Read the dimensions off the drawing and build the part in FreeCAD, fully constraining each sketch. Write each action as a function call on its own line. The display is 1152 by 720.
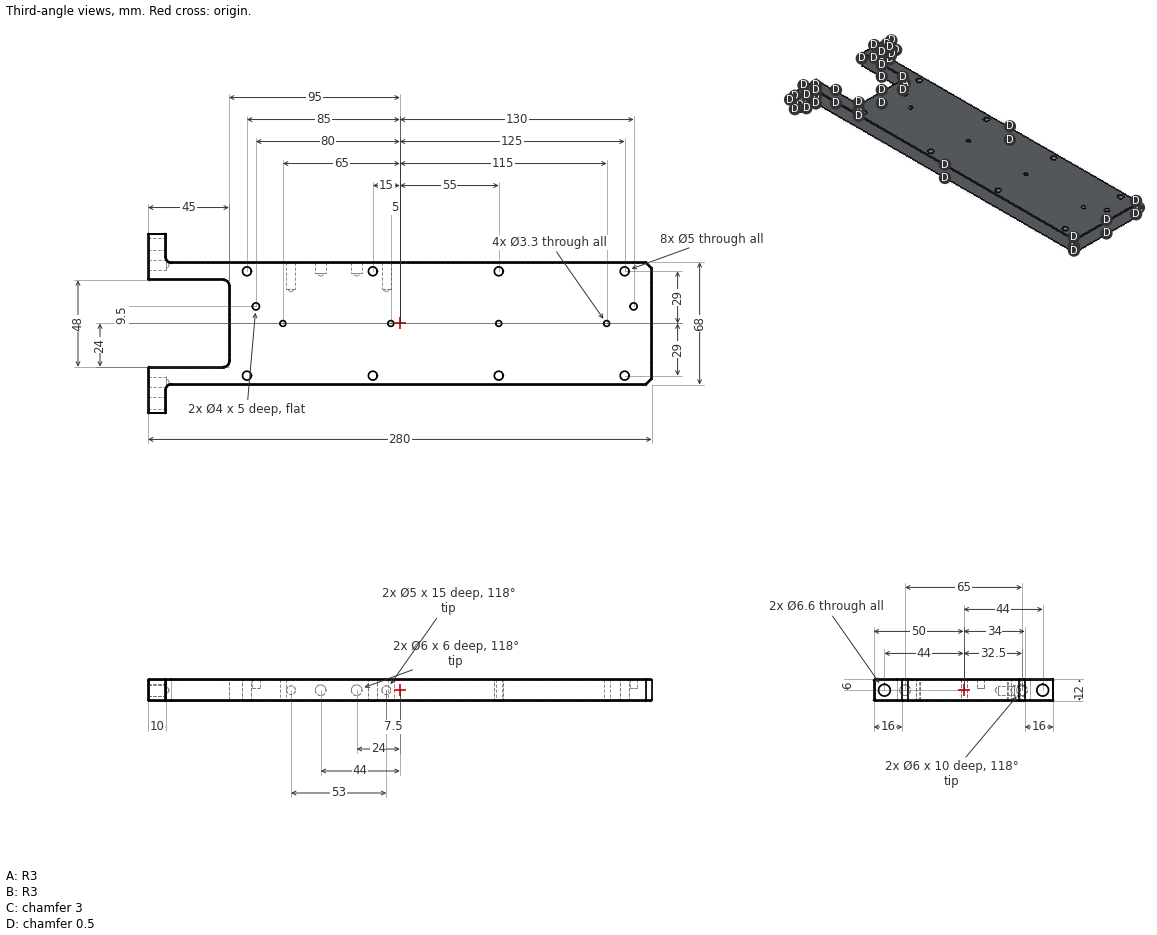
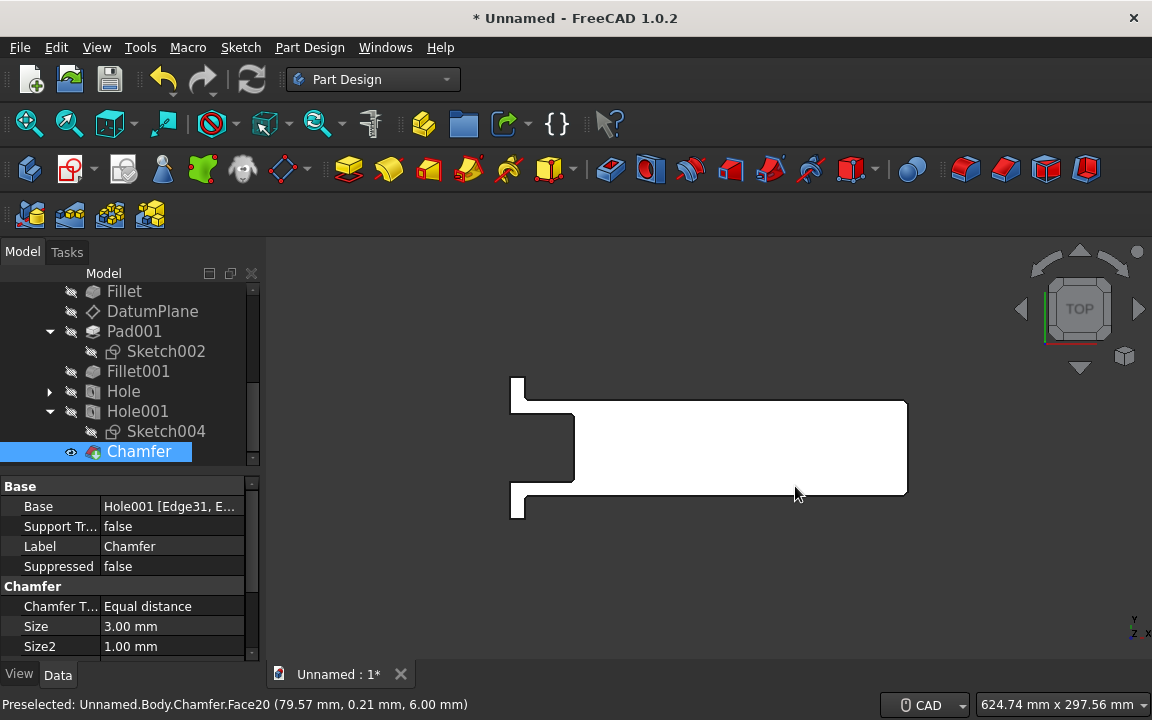
key(v)
key(f)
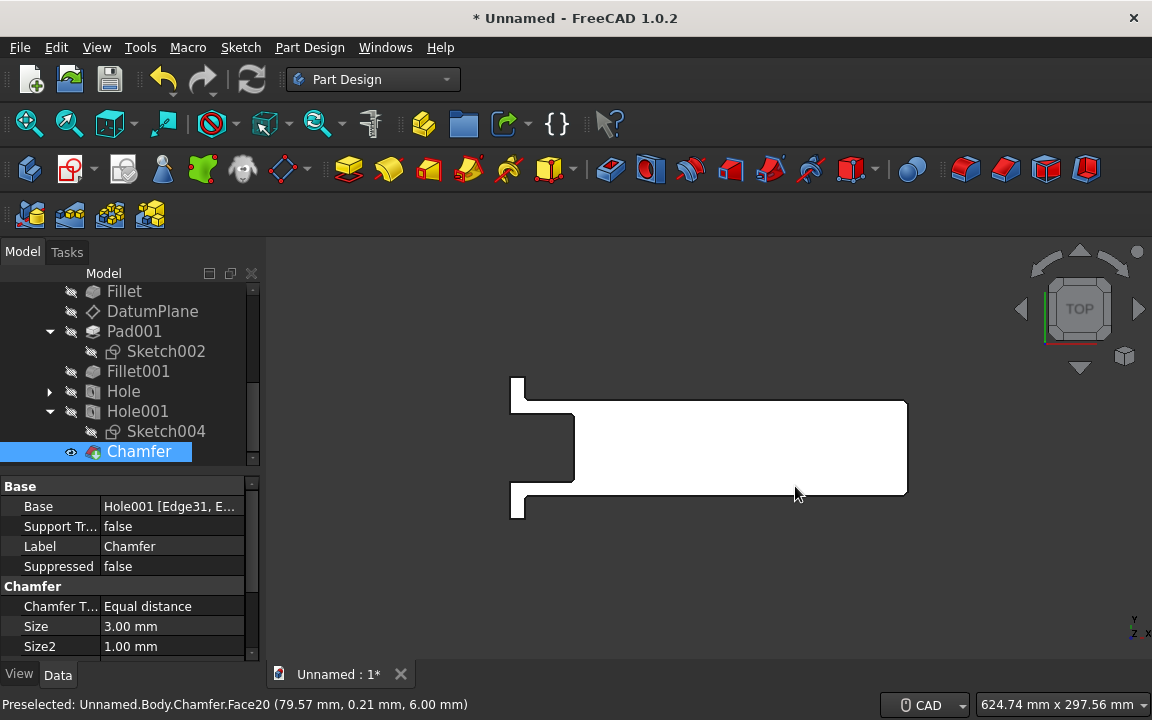
key(1)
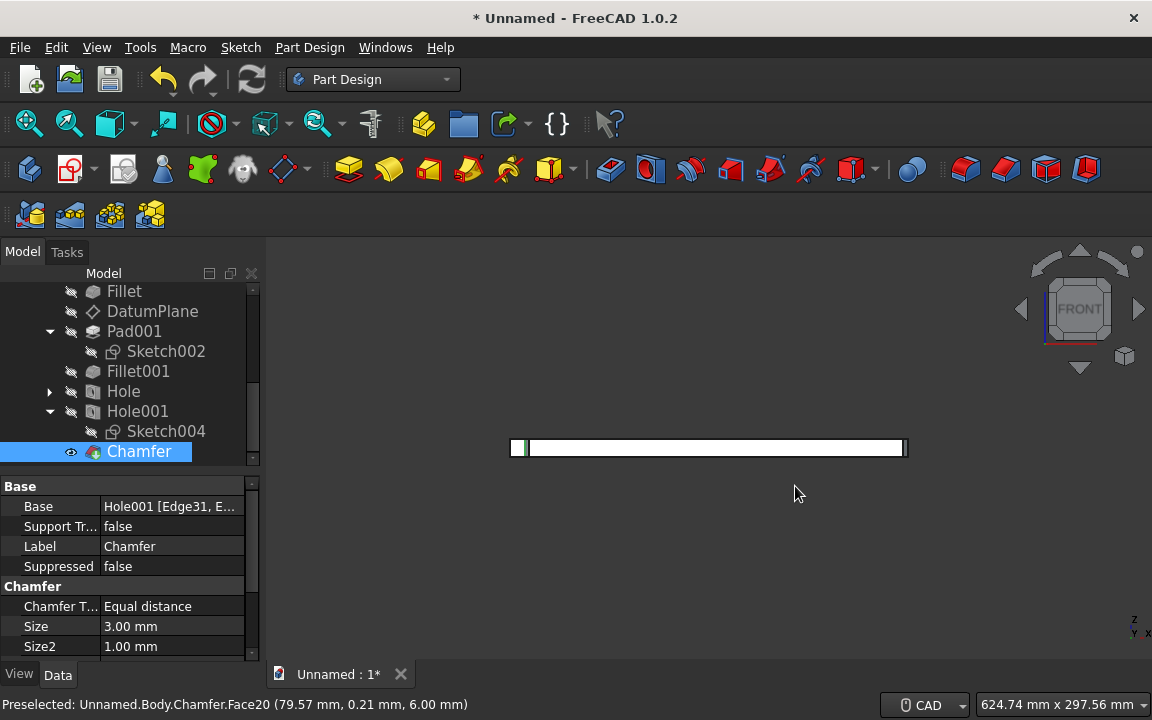
key(v)
key(f)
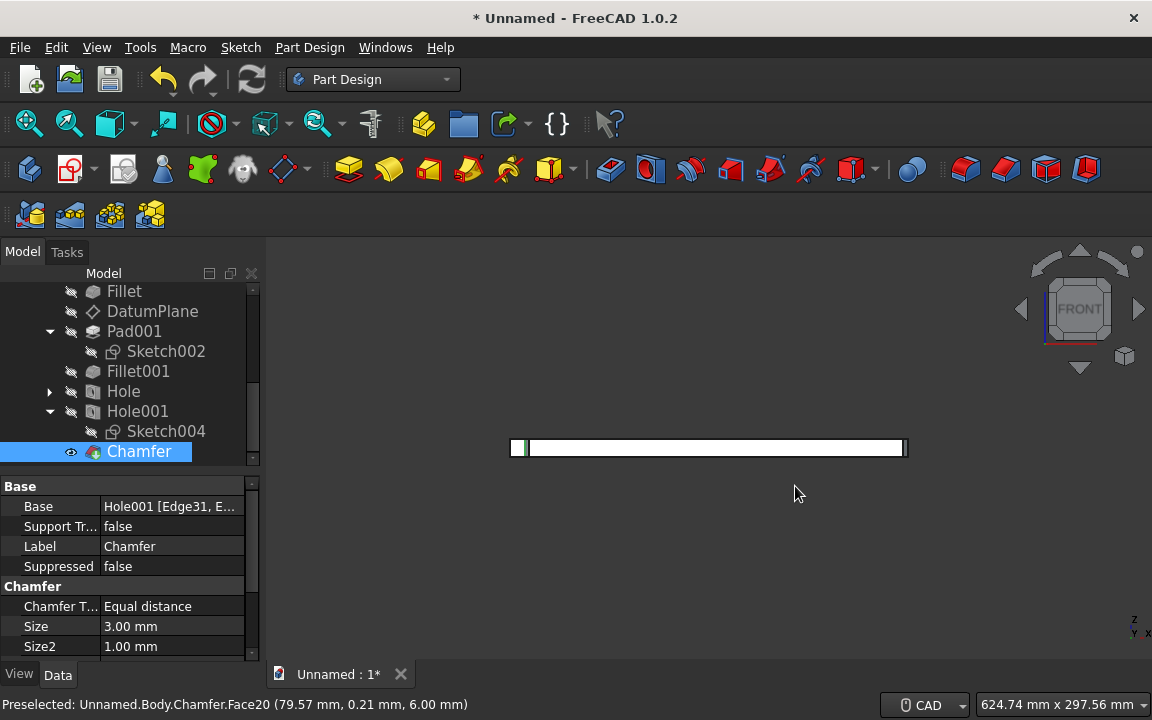
click(510, 447, ctrl)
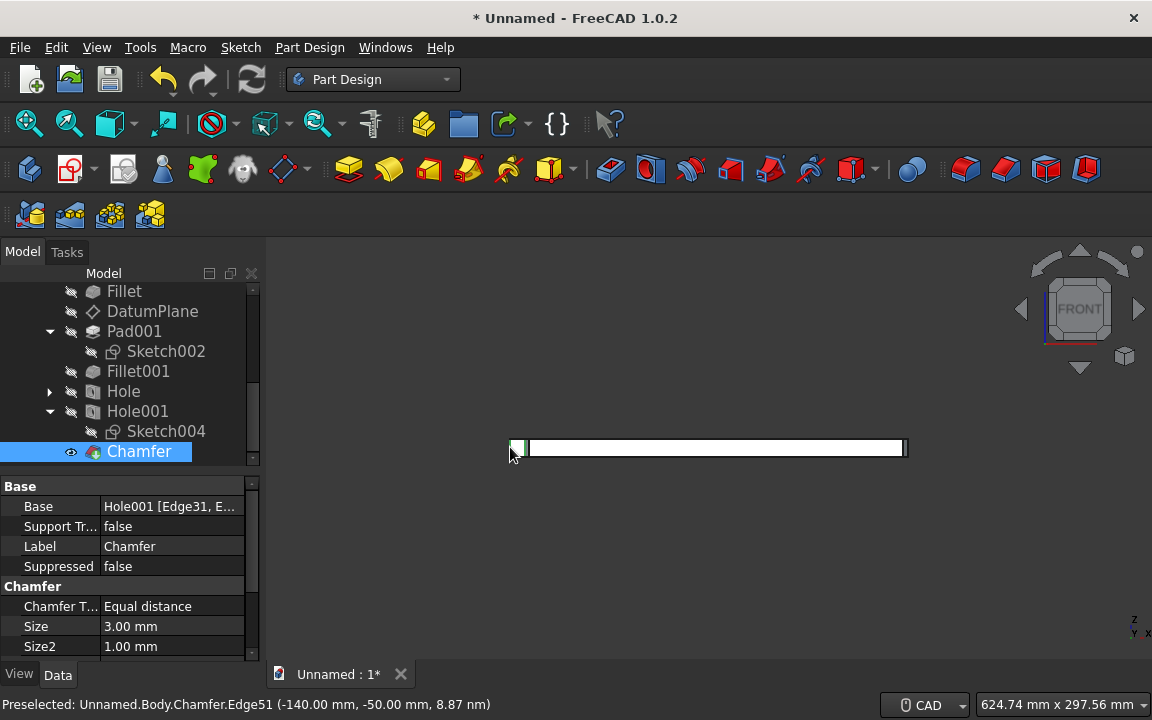
key(3)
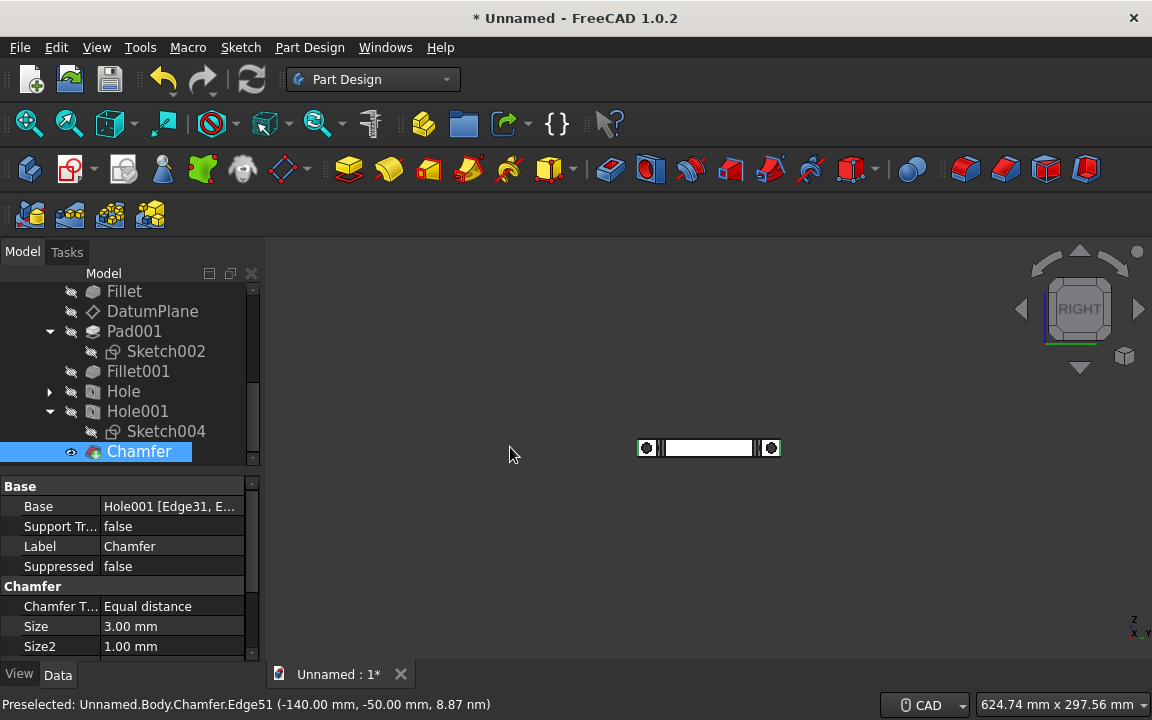
click(30, 124)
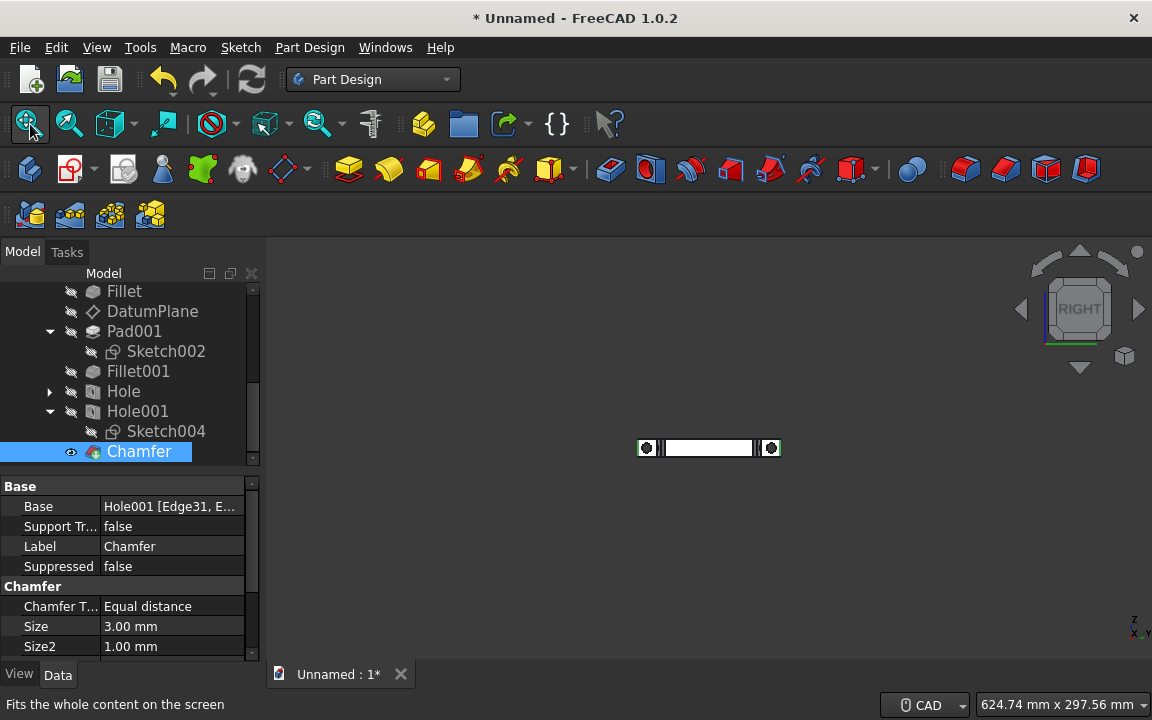
key(5)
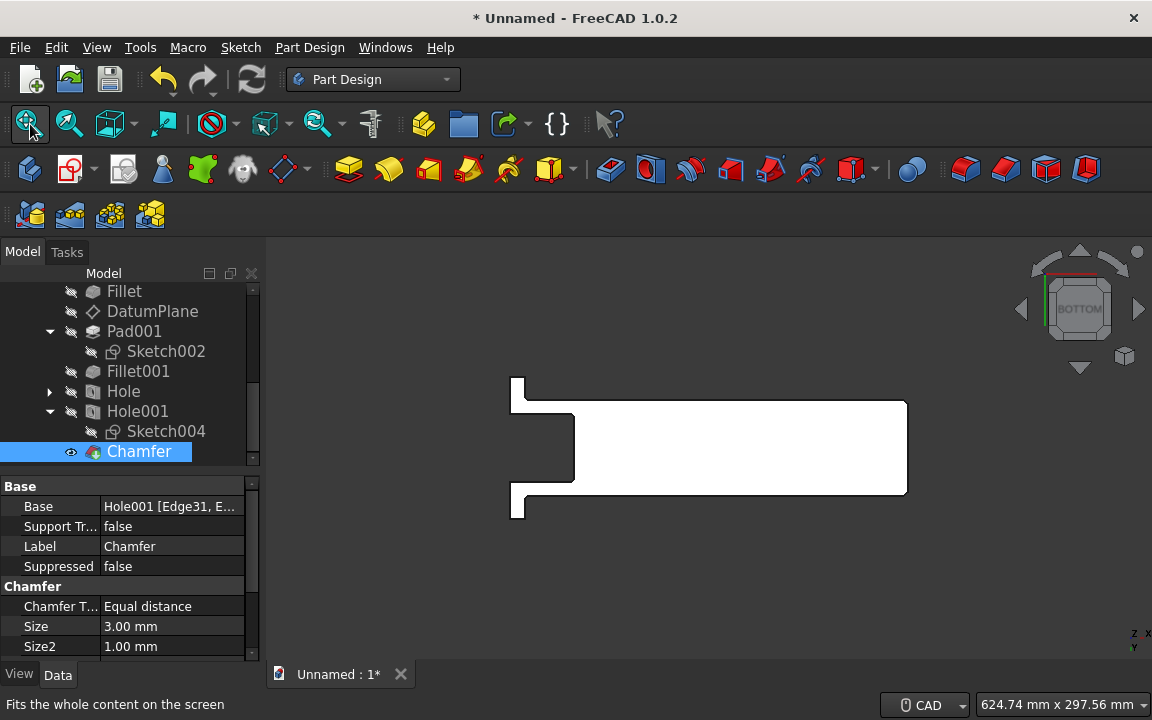
key(v)
key(f)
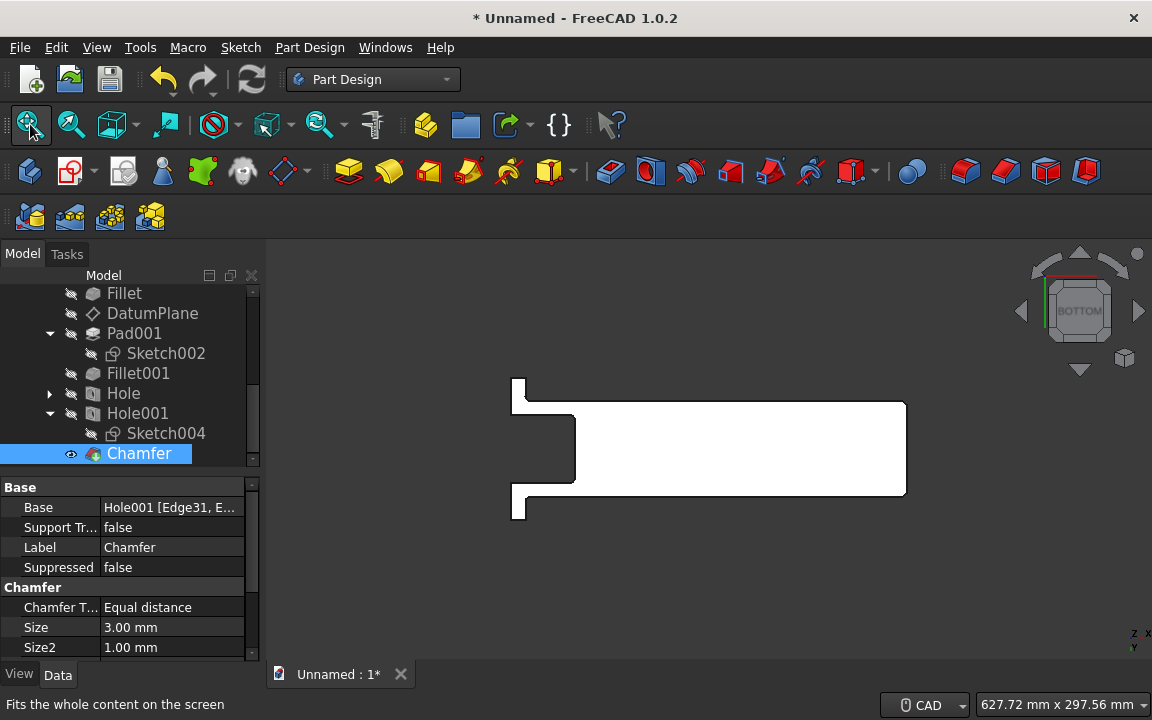
click(822, 448, ctrl)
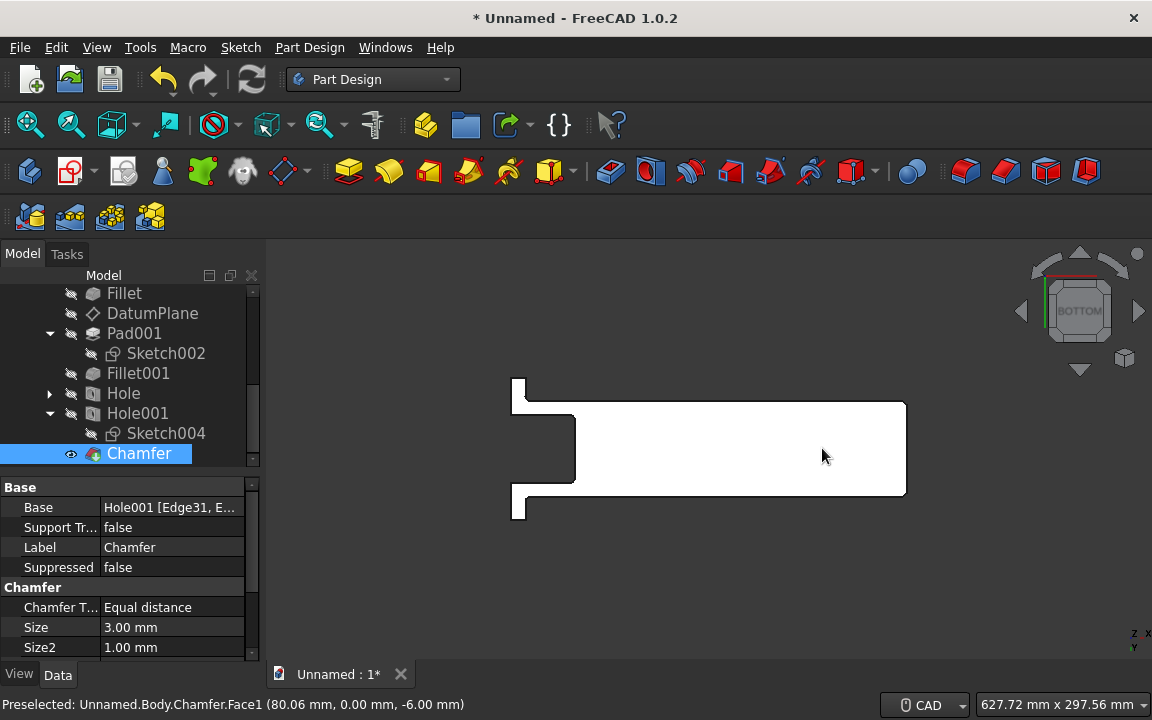
scroll(511, 482, up, 5)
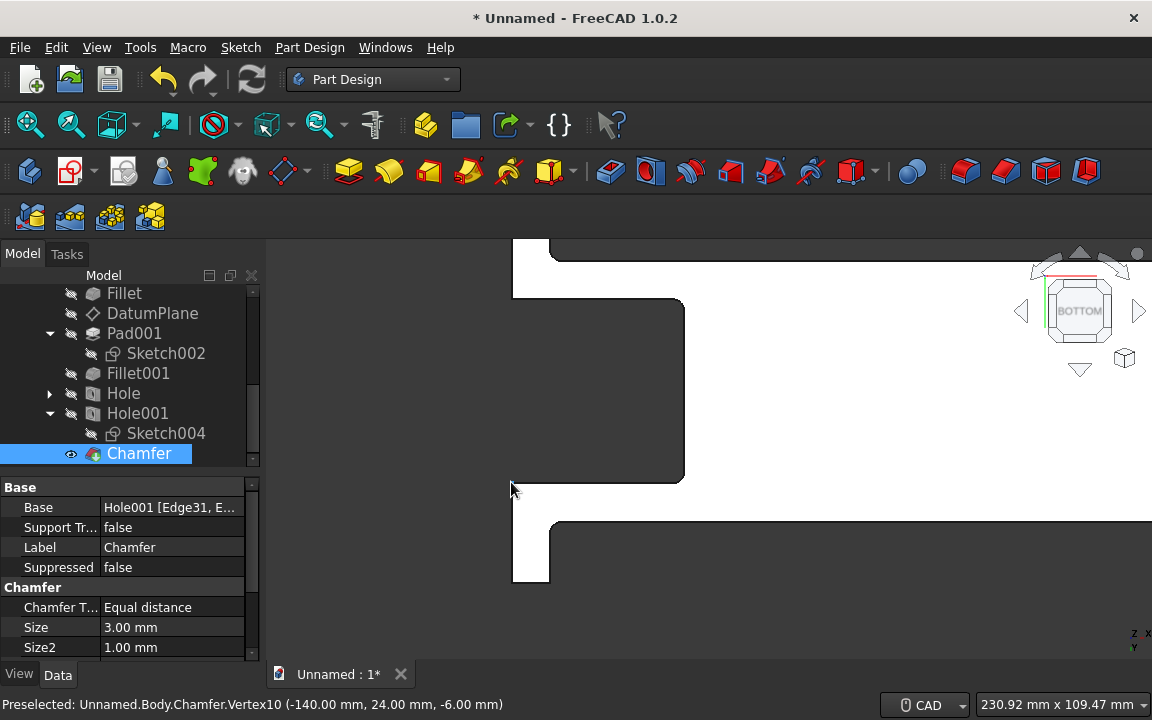
key(v)
key(f)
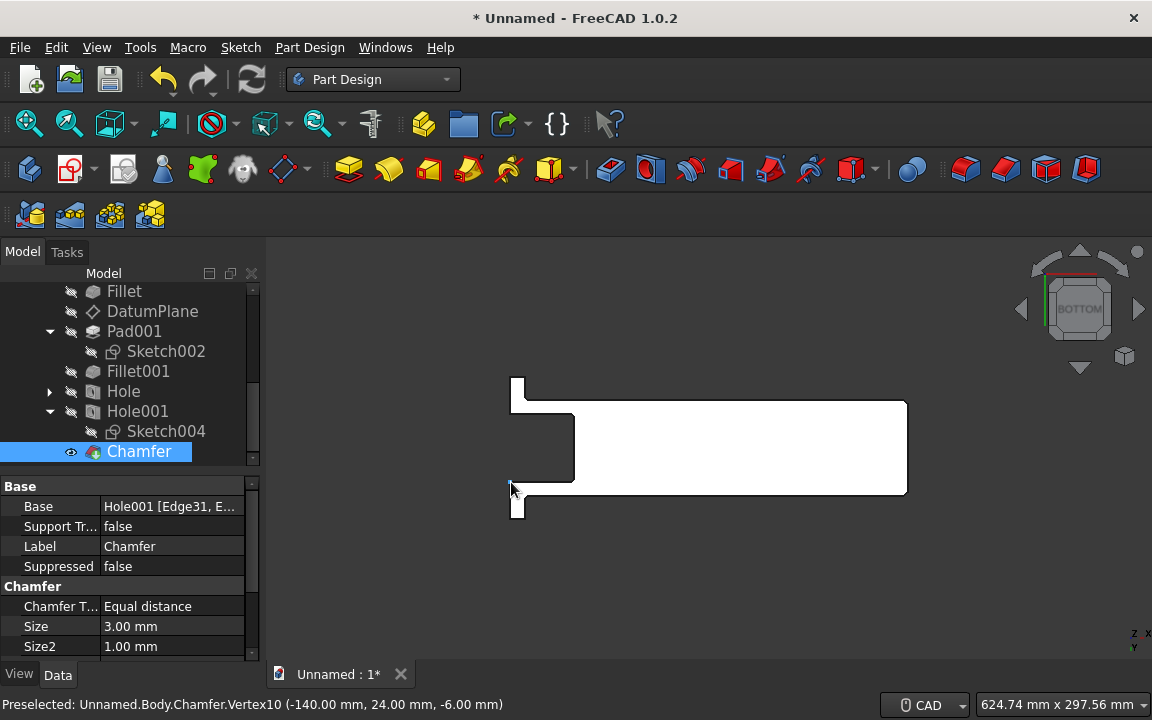
key(4)